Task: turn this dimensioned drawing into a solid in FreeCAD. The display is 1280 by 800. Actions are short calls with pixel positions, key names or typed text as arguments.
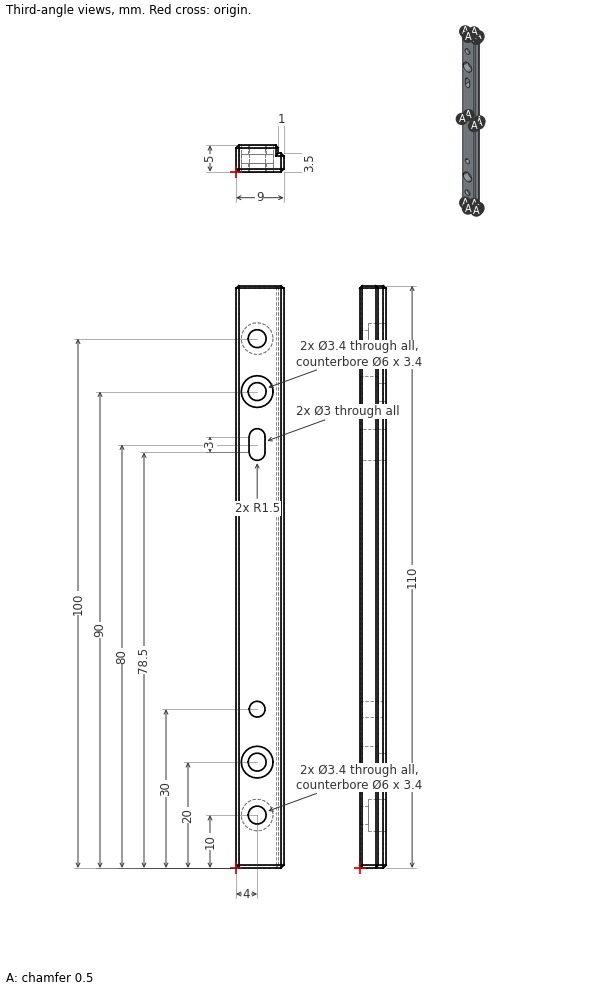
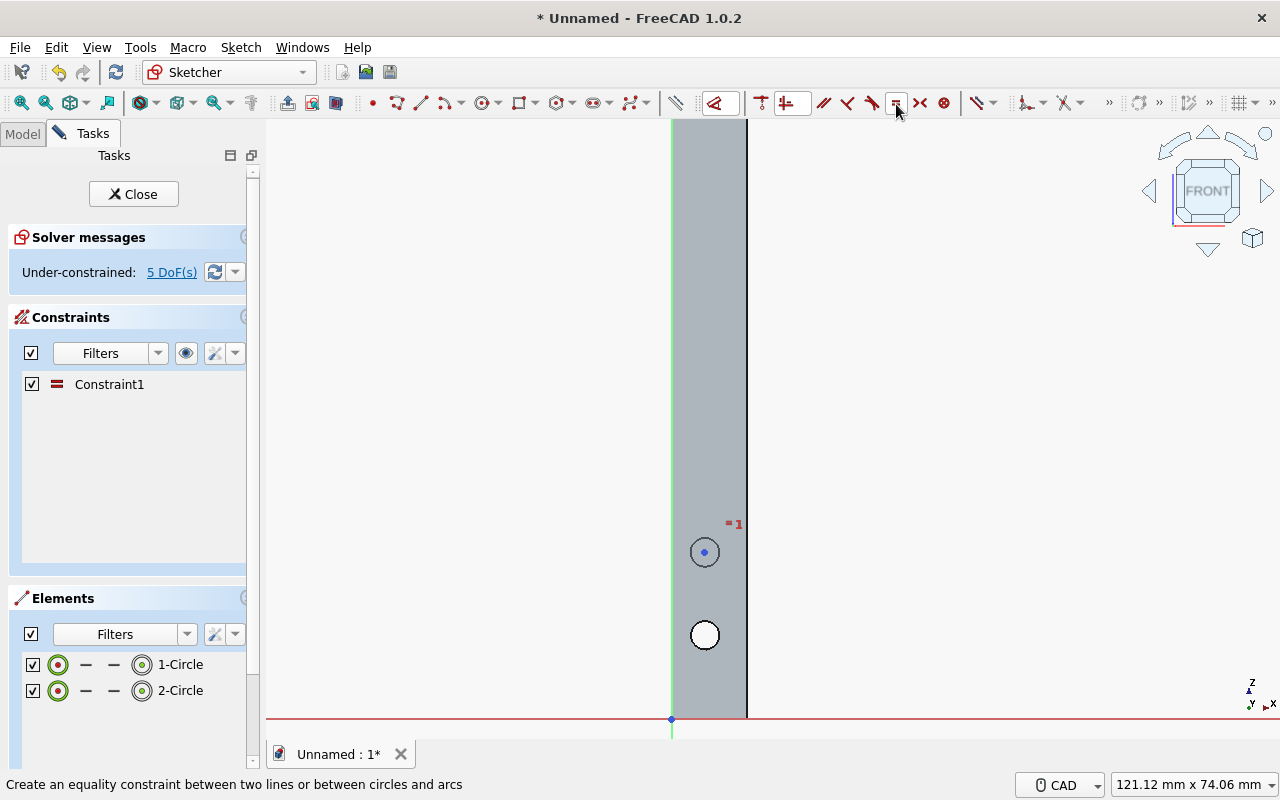
scroll(715, 543, down, 3)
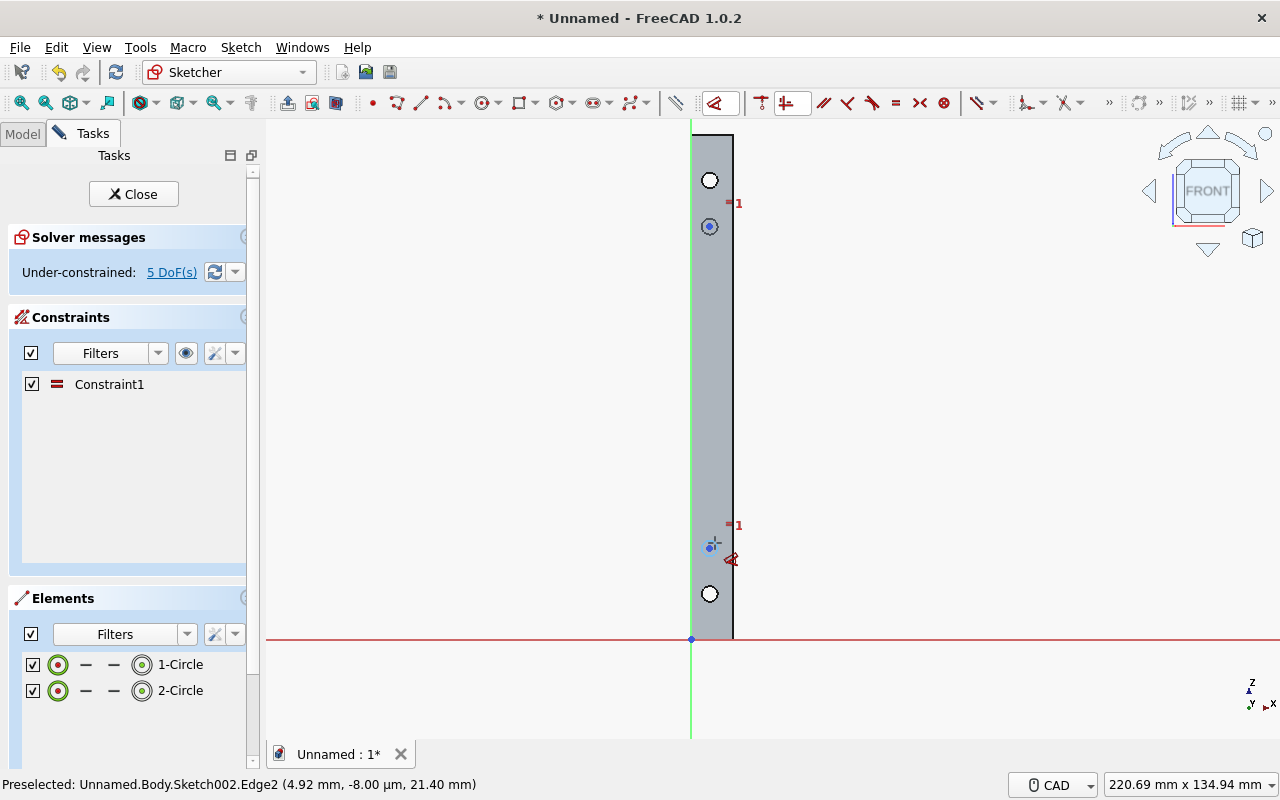
scroll(715, 221, up, 5)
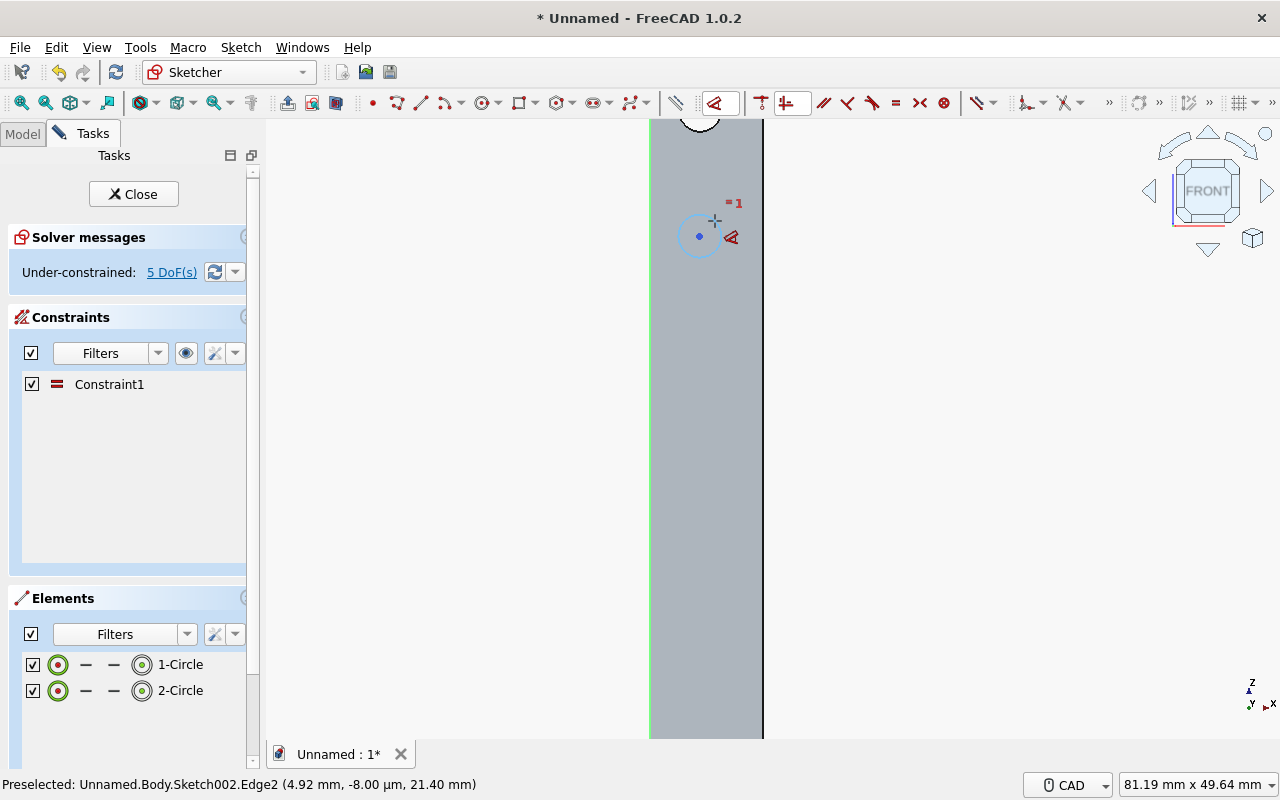
click(715, 221)
click(738, 198)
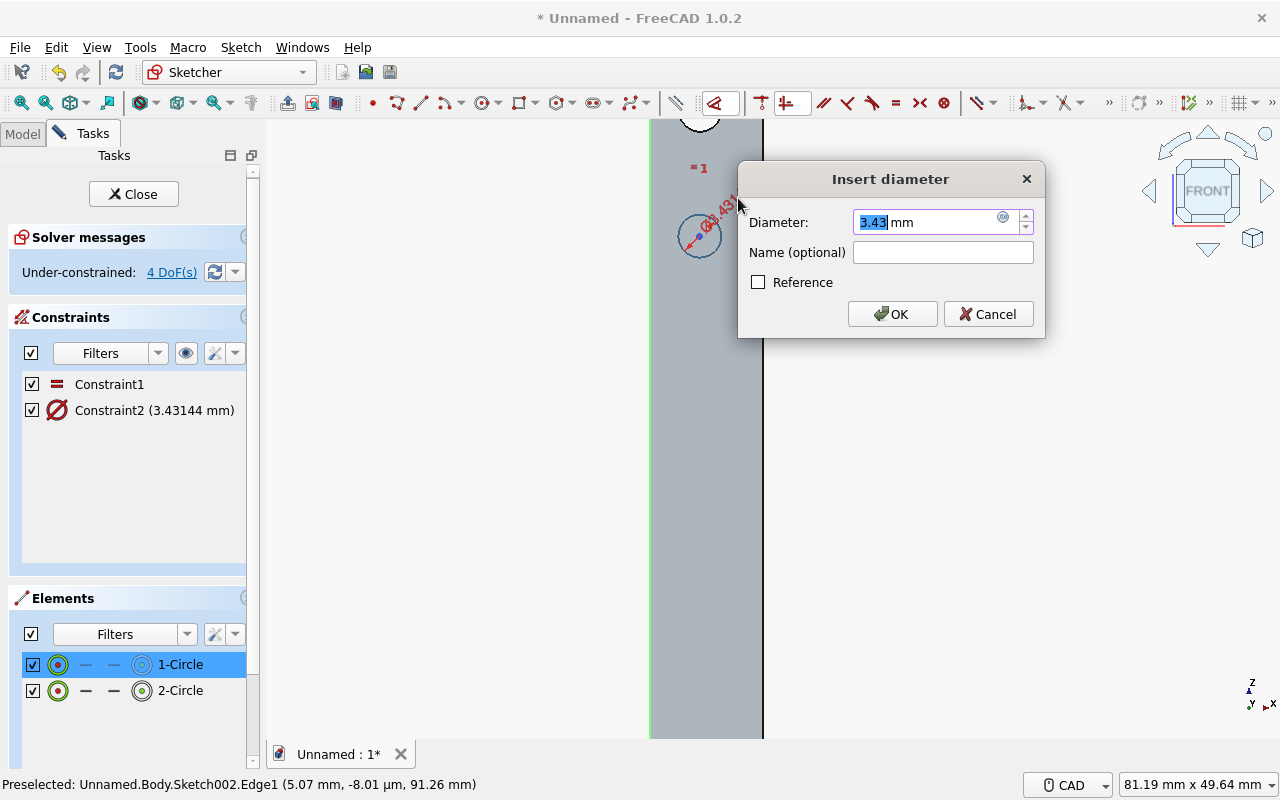
text(3.4)
key(Return)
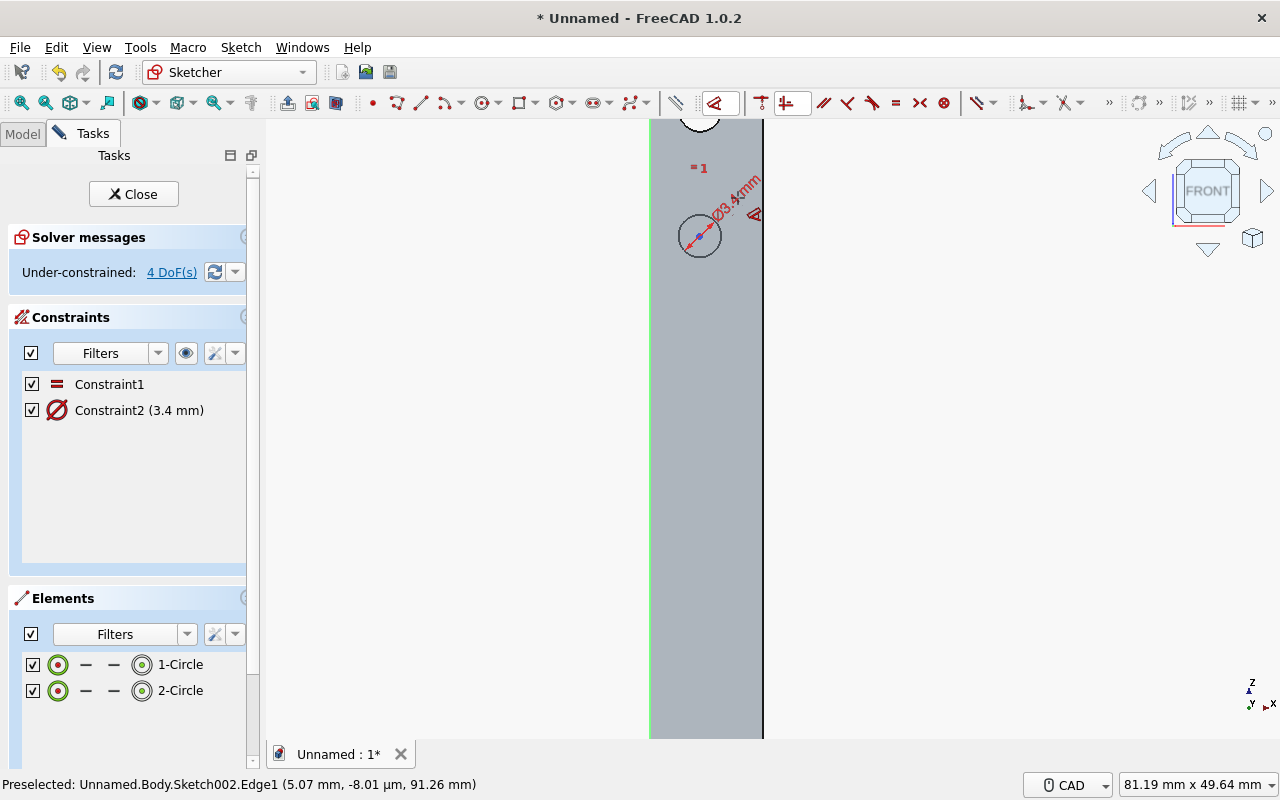
click(700, 236)
click(664, 202)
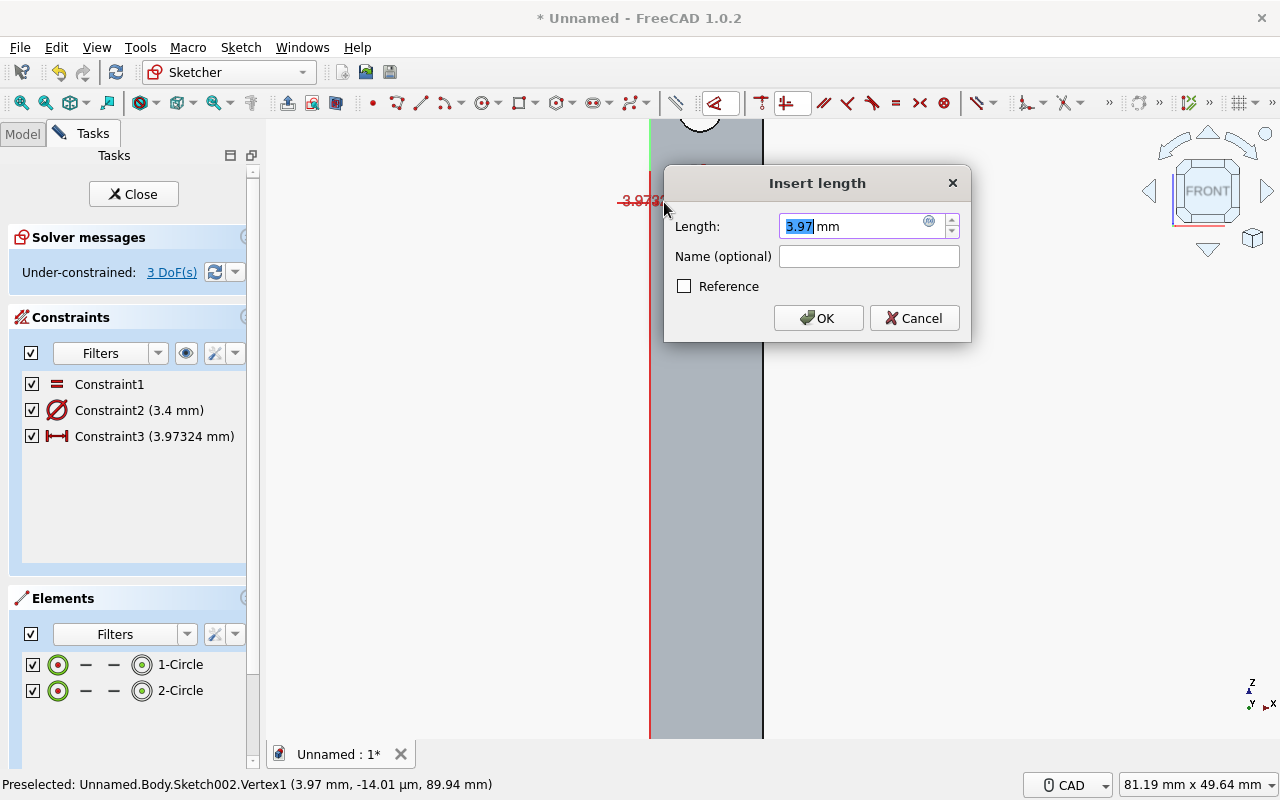
text(4)
key(Return)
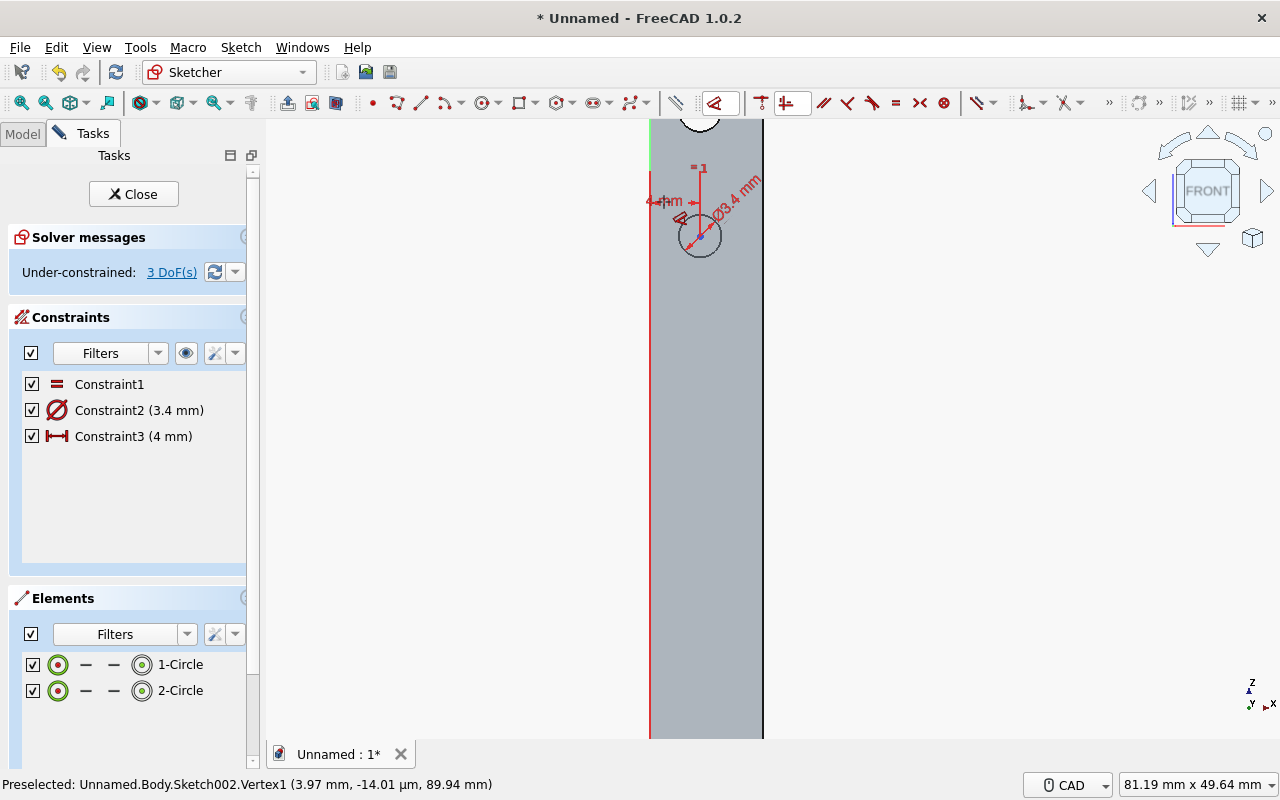
scroll(715, 221, down, 5)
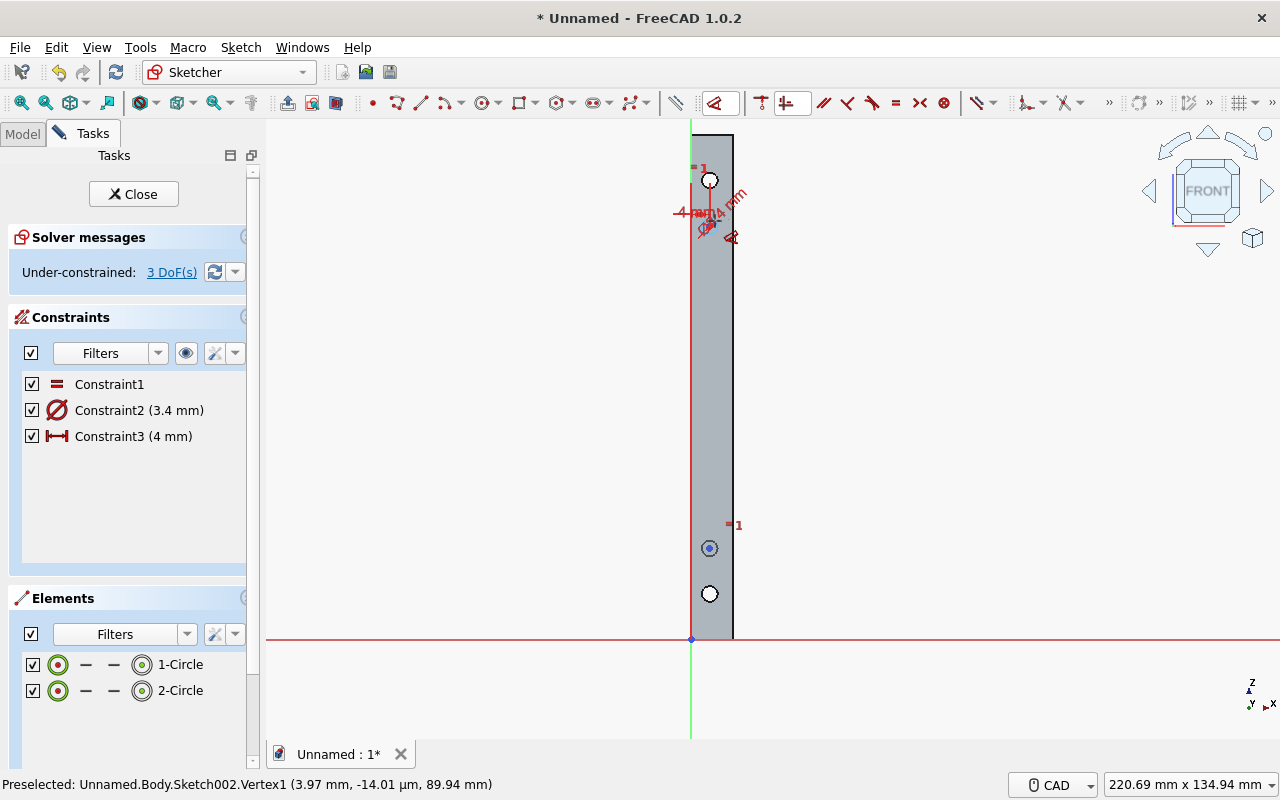
scroll(710, 548, up, 4)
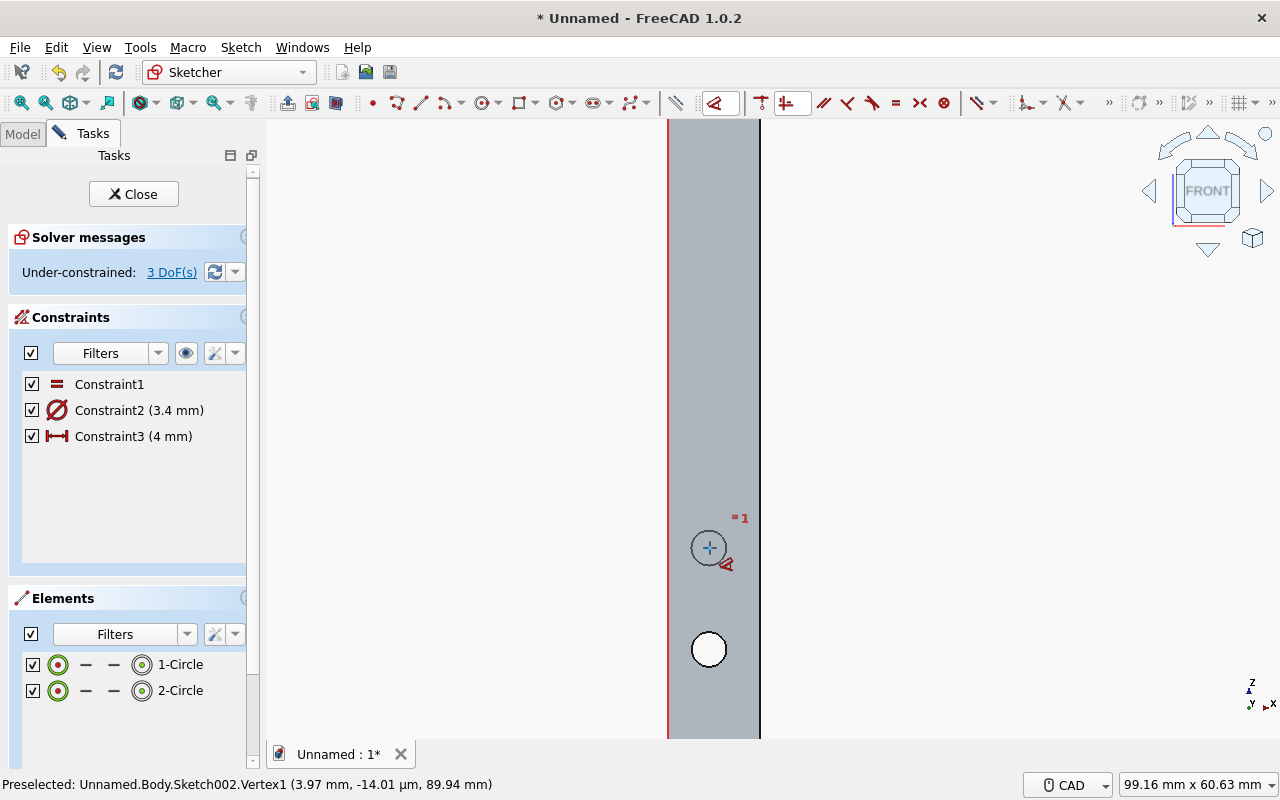
click(709, 548)
click(688, 514)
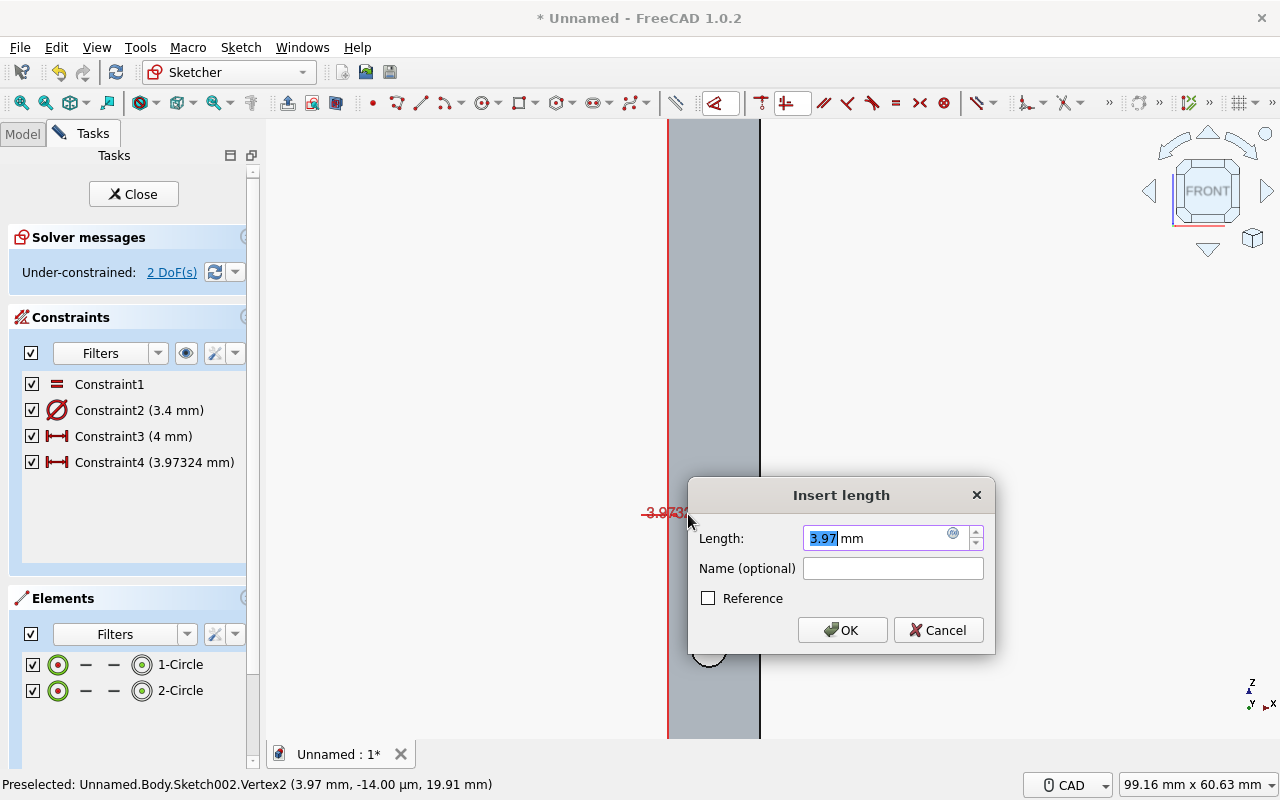
text(4)
key(Return)